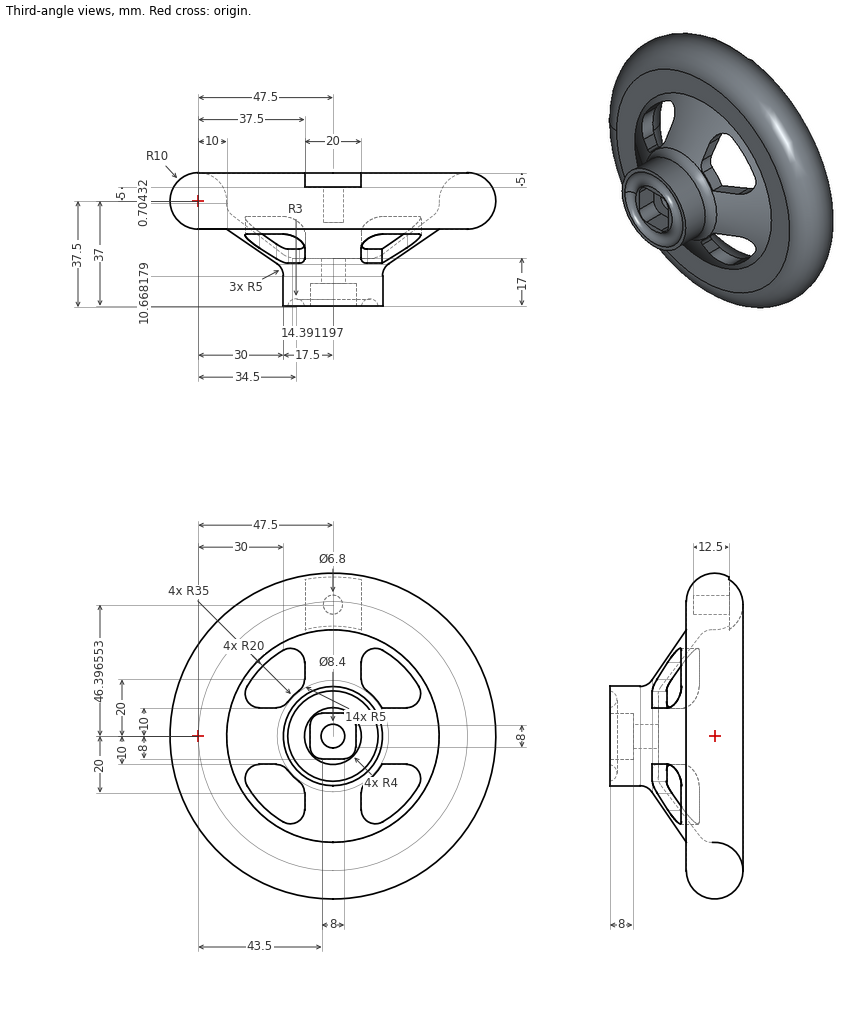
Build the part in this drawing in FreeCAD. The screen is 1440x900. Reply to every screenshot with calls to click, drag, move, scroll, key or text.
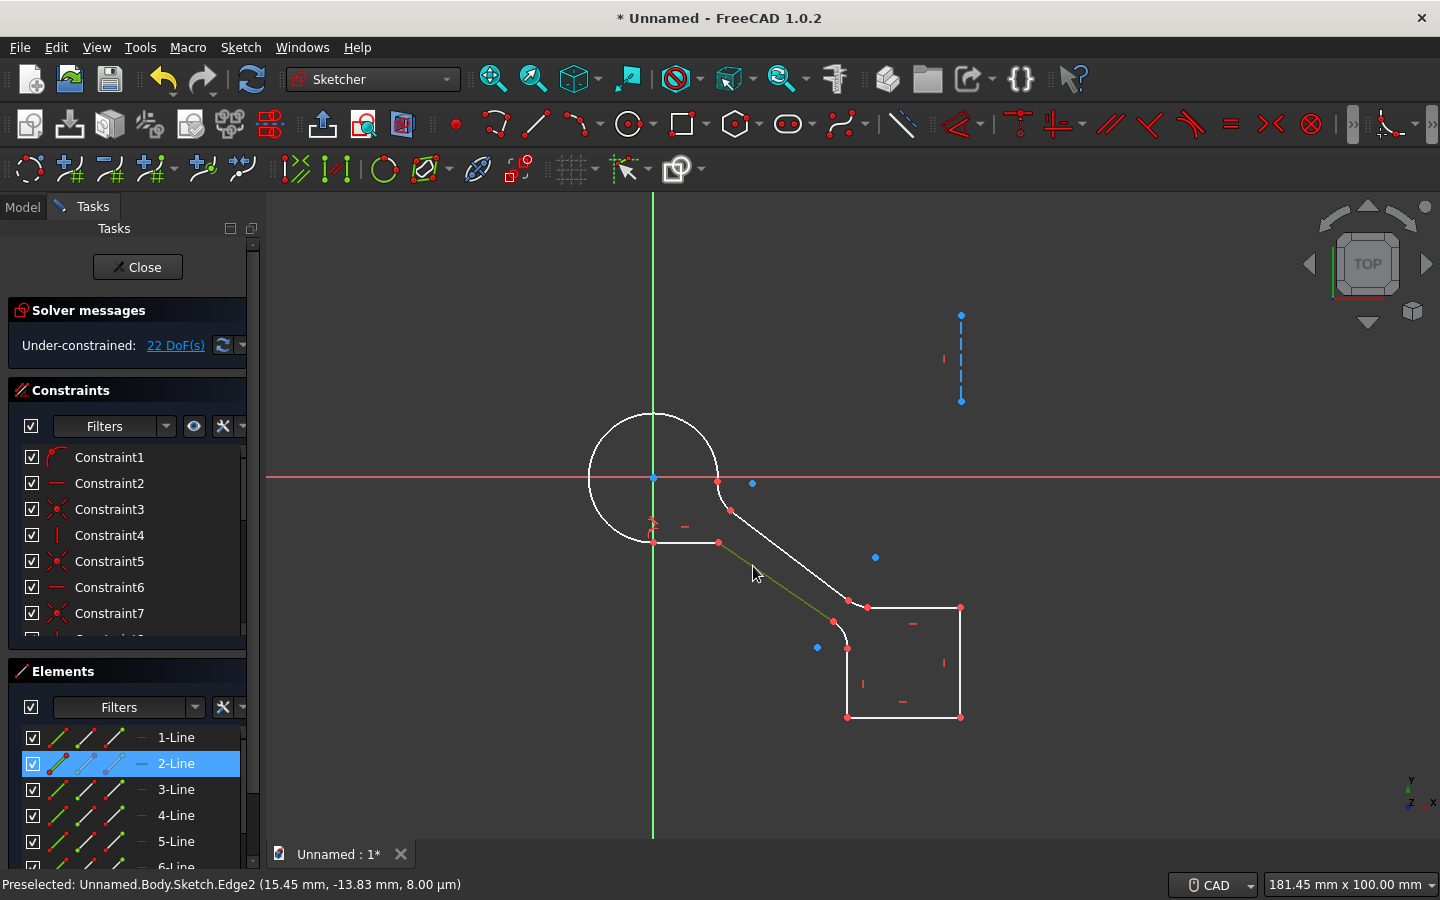
scroll(846, 639, up, 2)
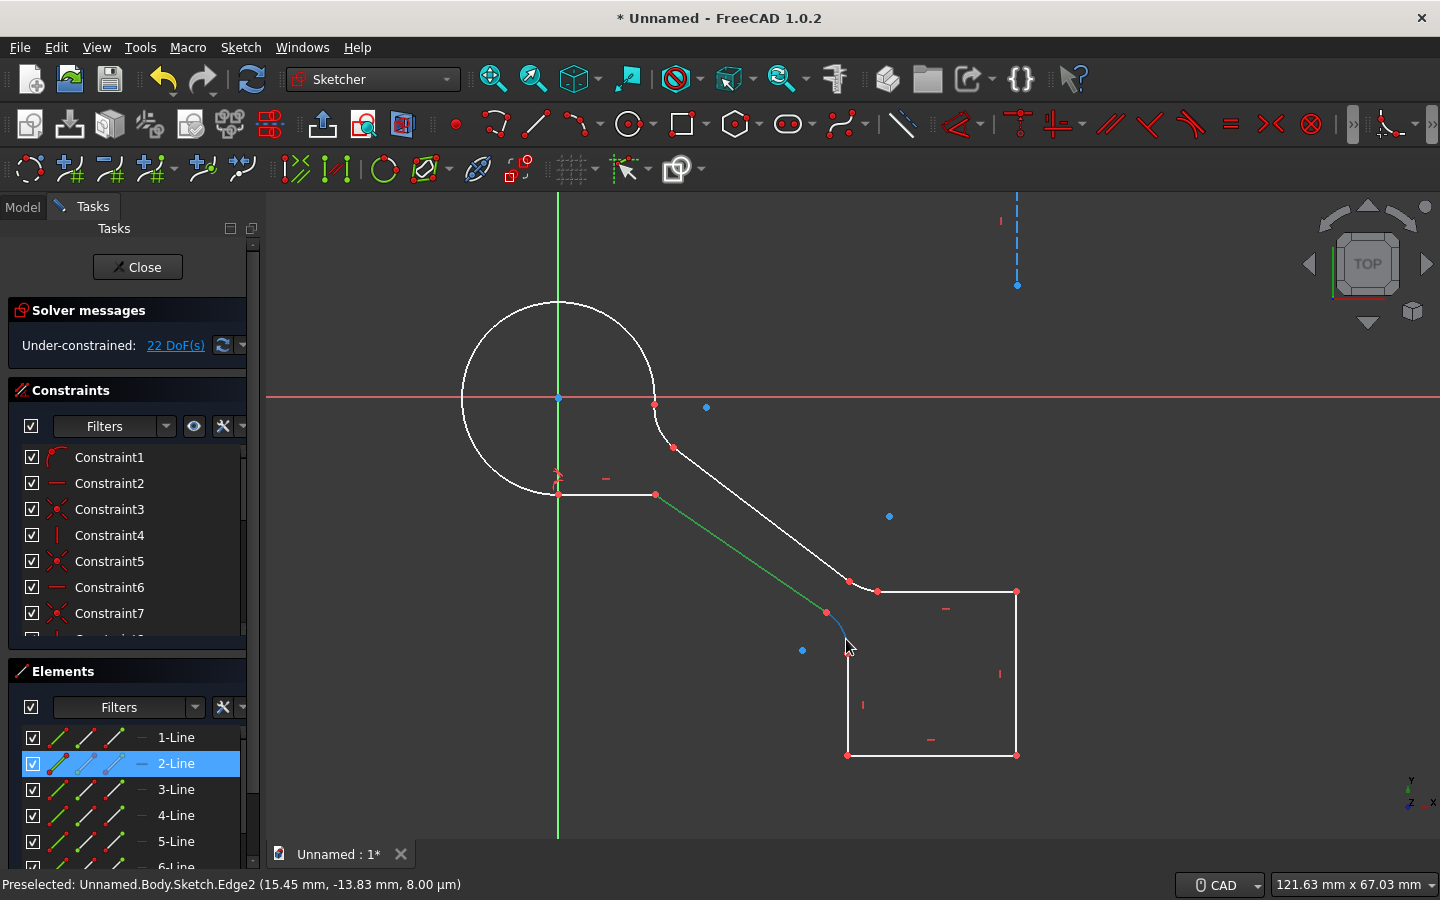
click(846, 639)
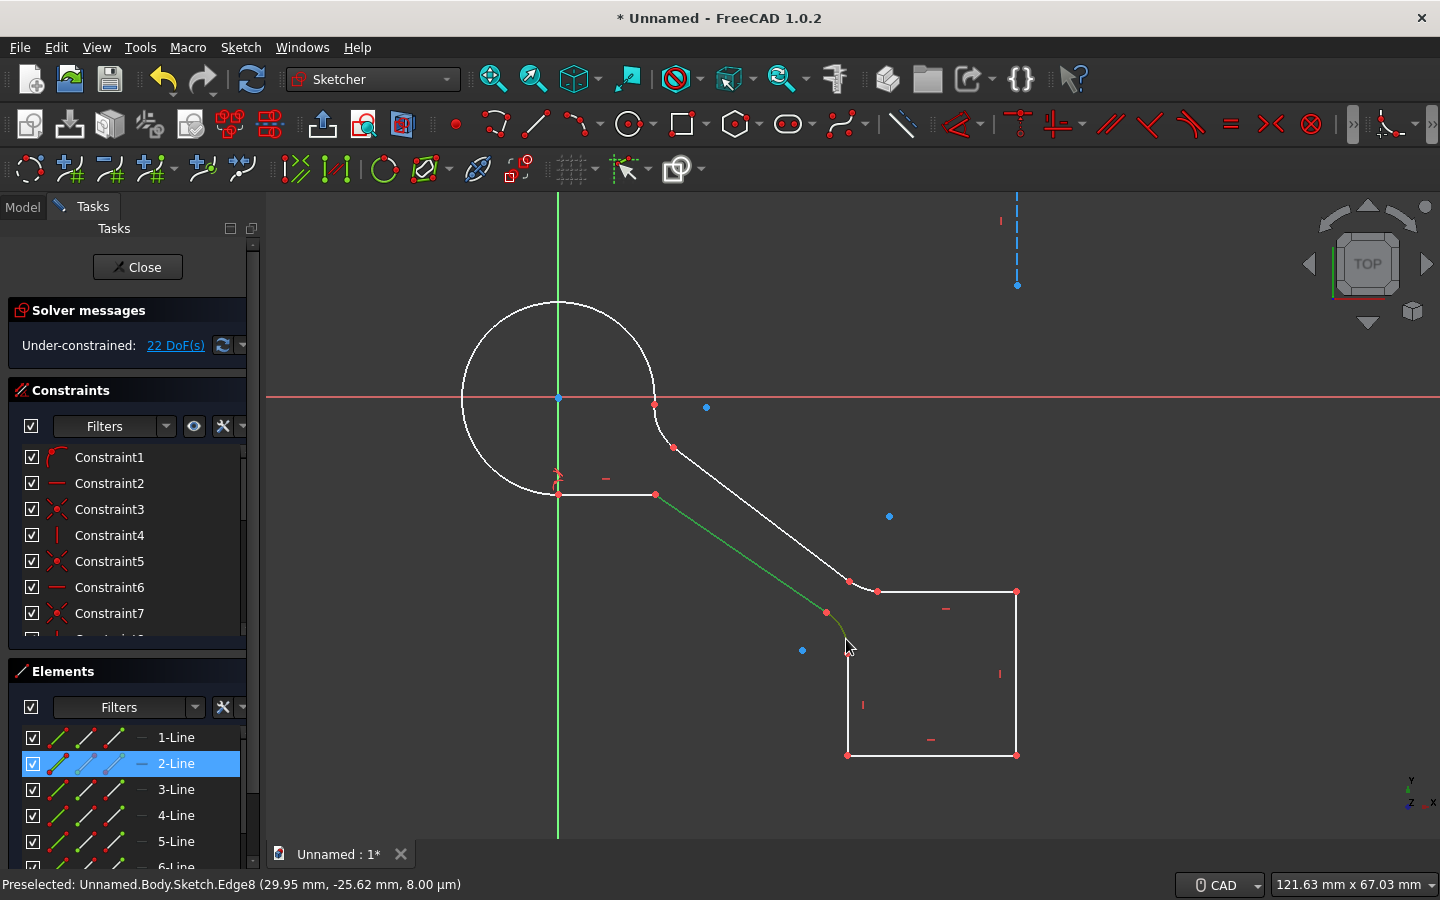
click(1192, 124)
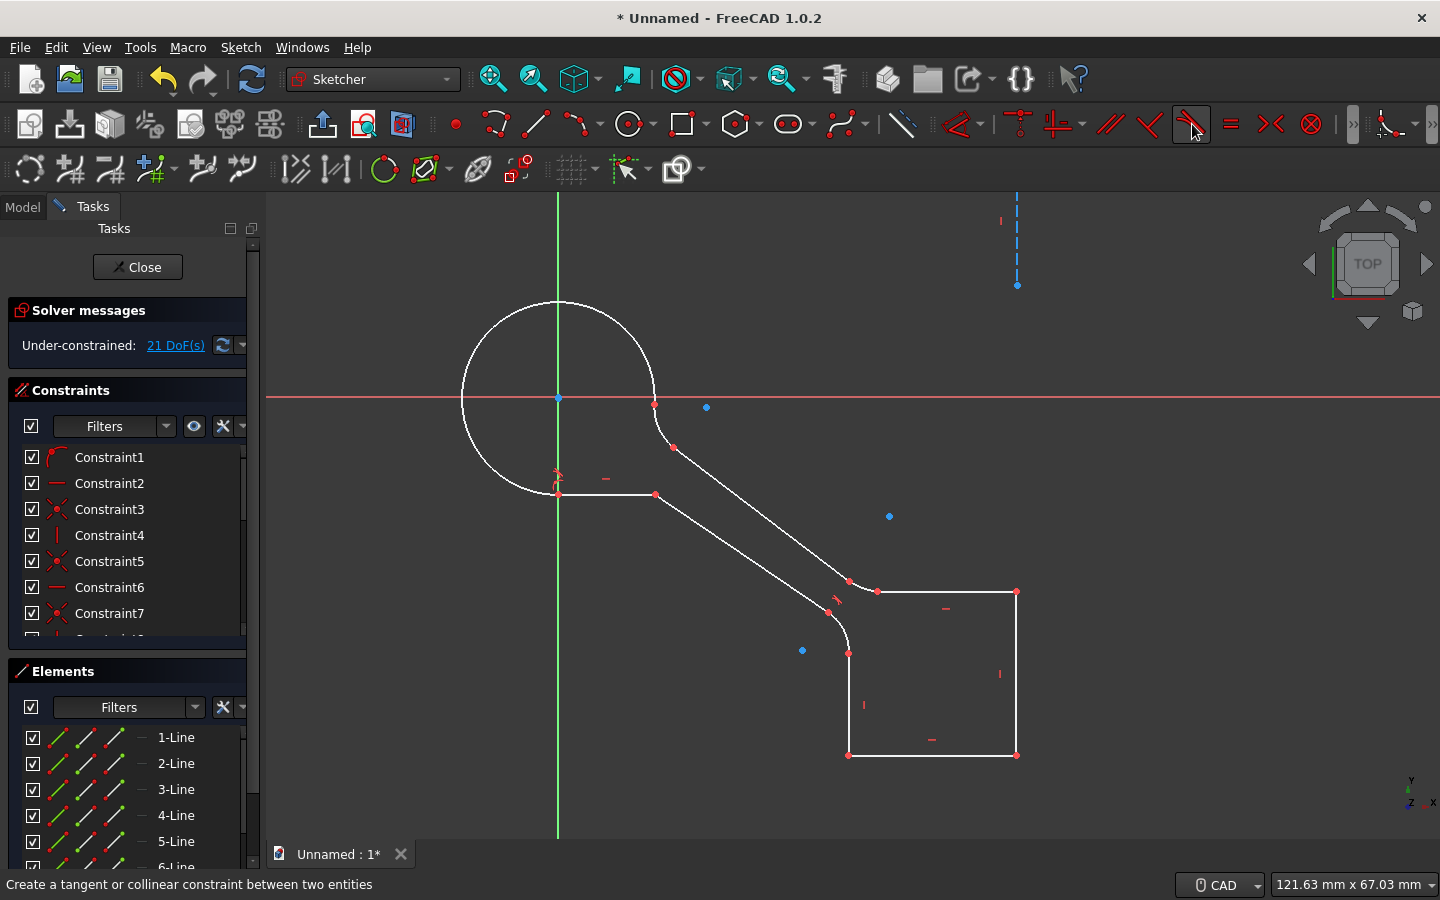
click(849, 684)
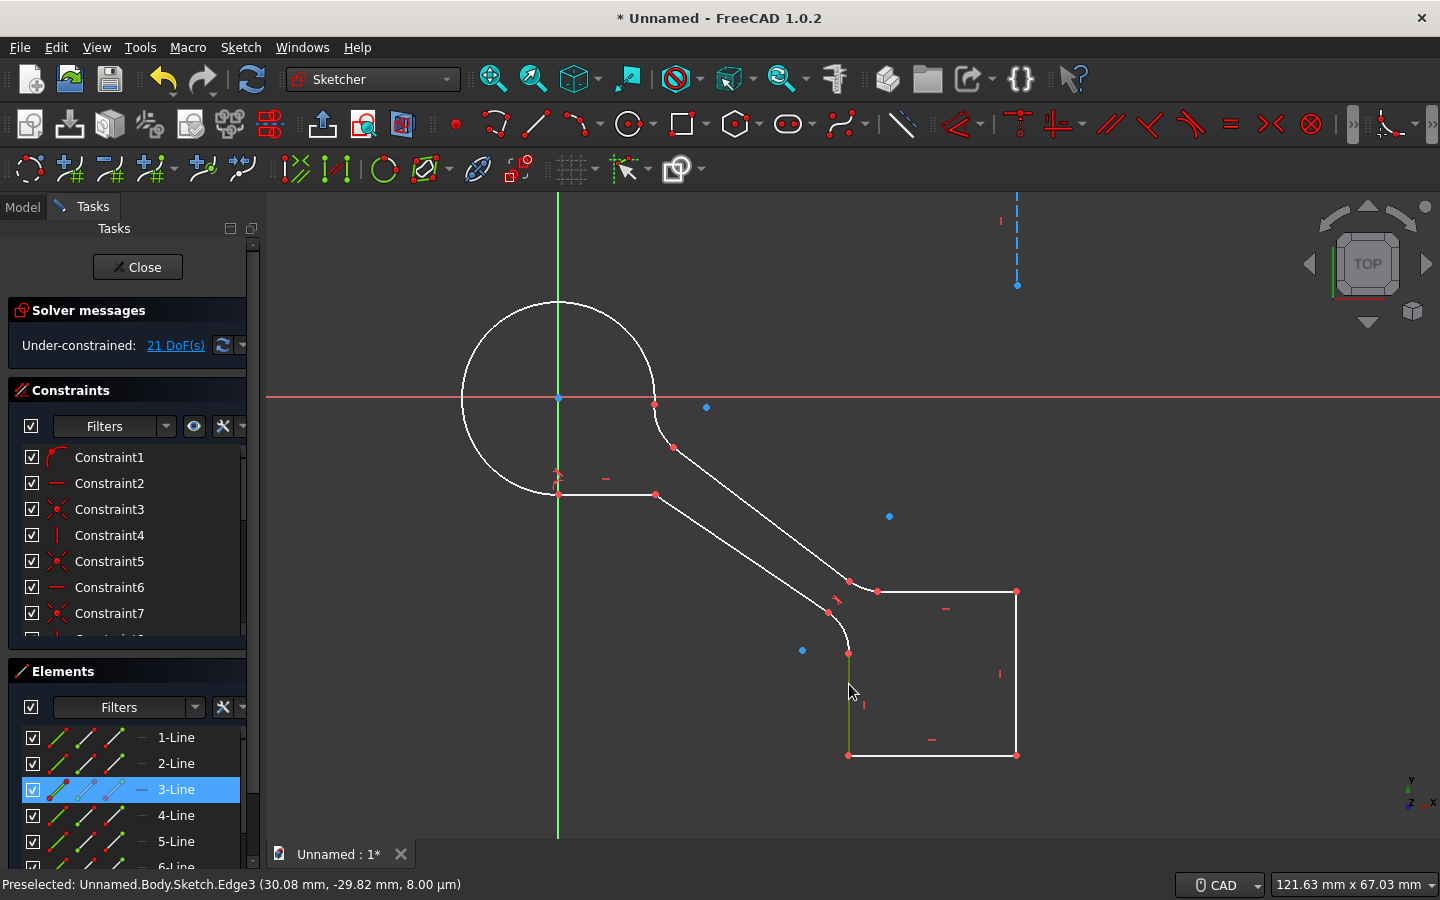
click(847, 639)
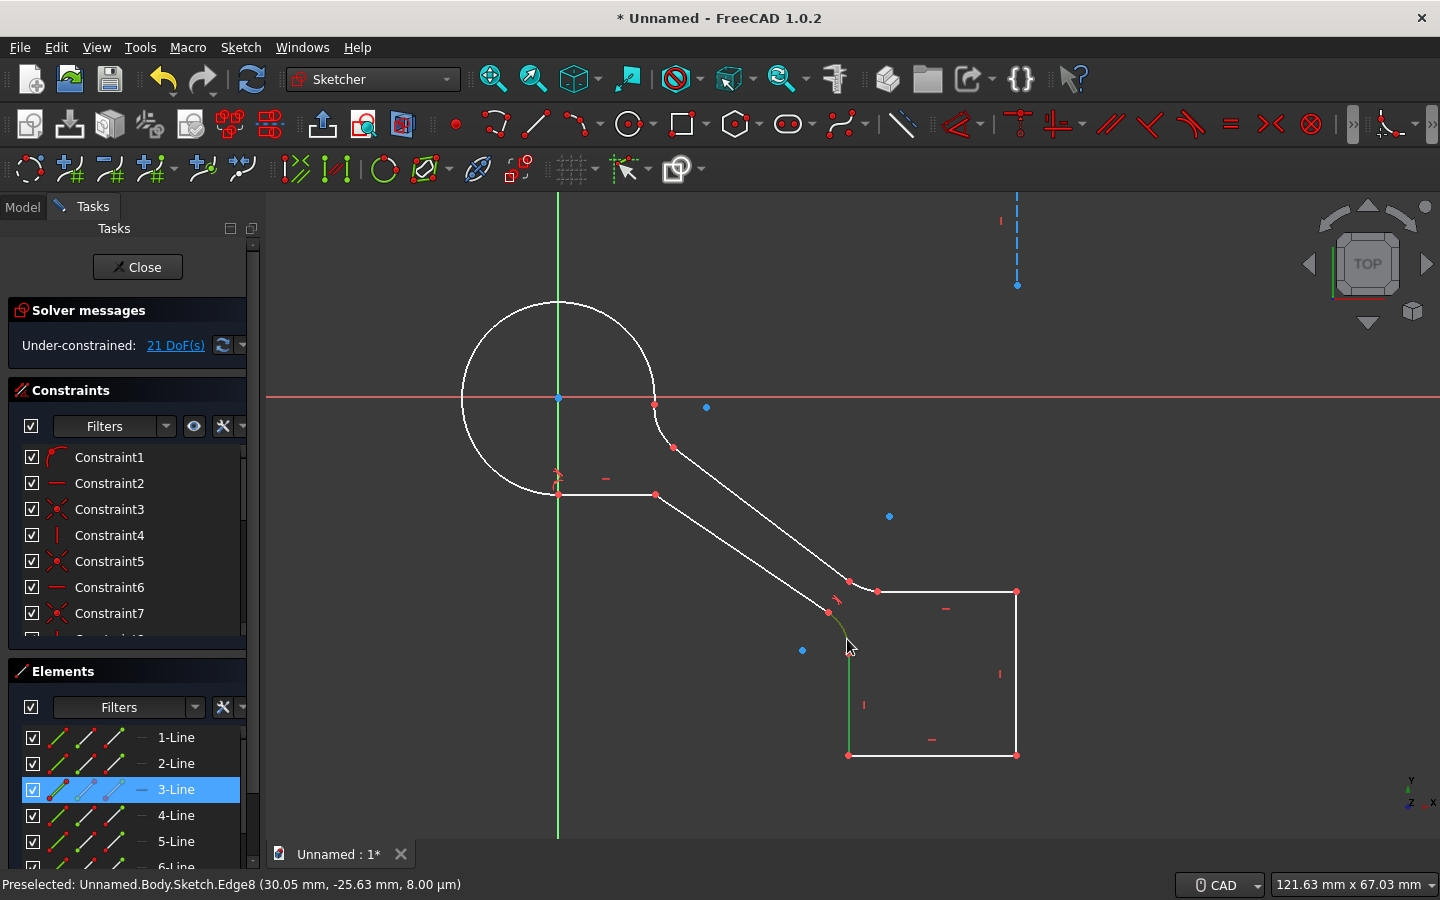
click(1192, 124)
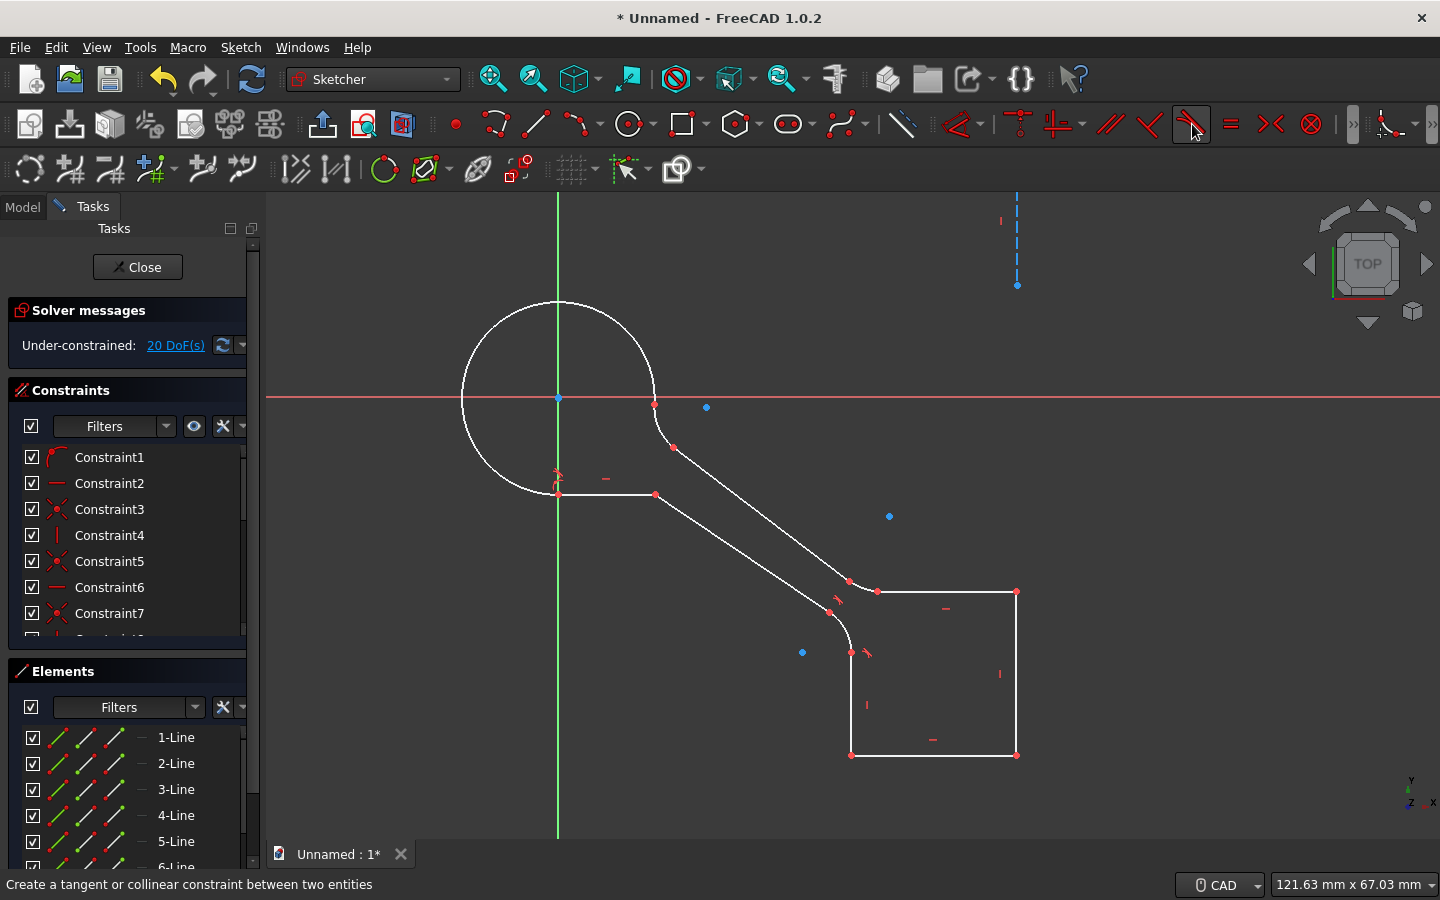
click(975, 592)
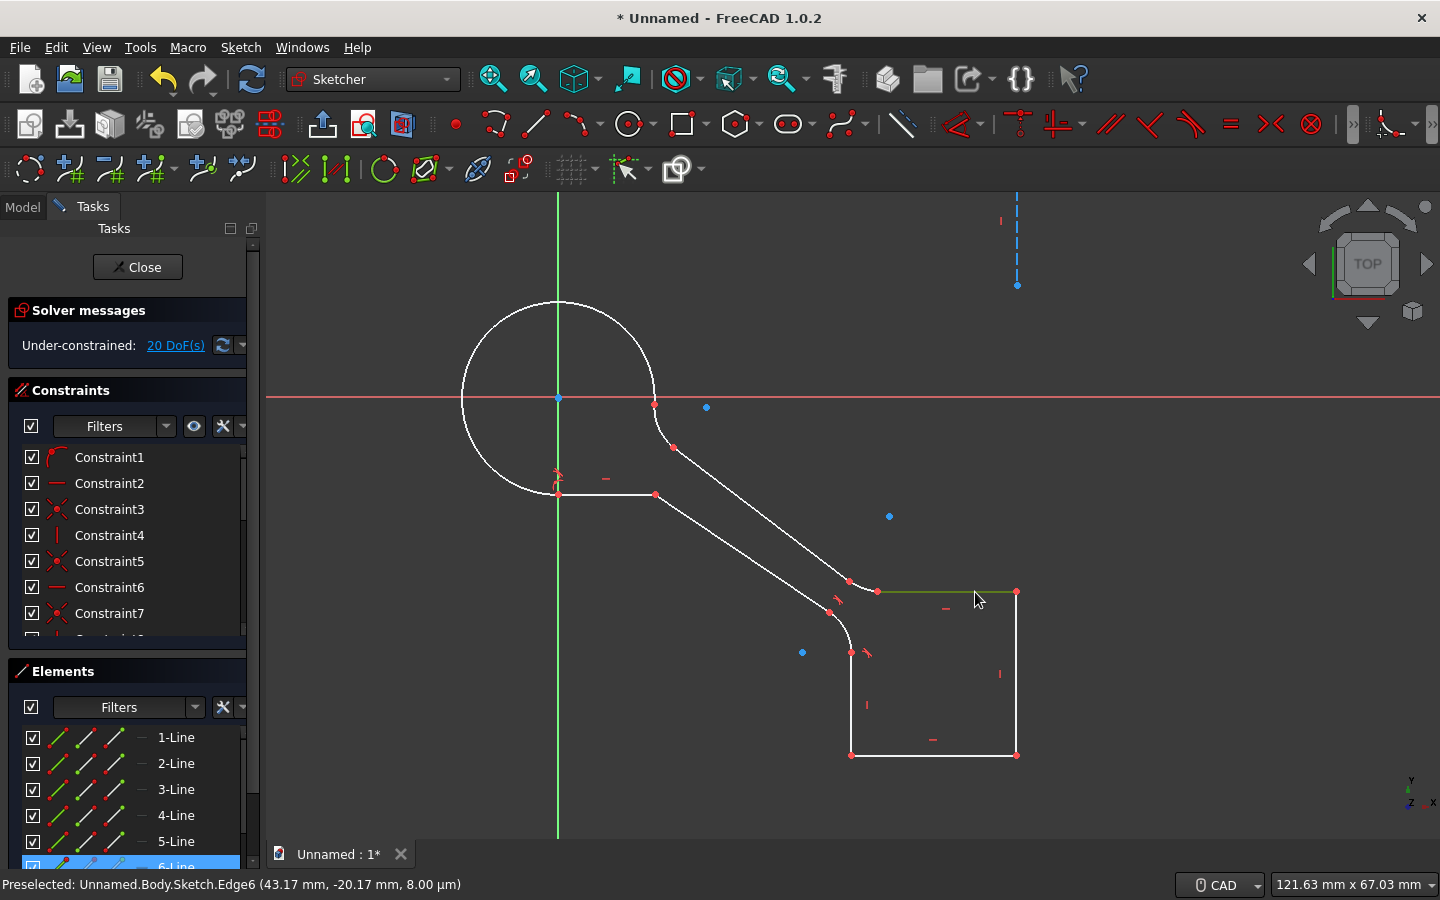
scroll(857, 586, up, 3)